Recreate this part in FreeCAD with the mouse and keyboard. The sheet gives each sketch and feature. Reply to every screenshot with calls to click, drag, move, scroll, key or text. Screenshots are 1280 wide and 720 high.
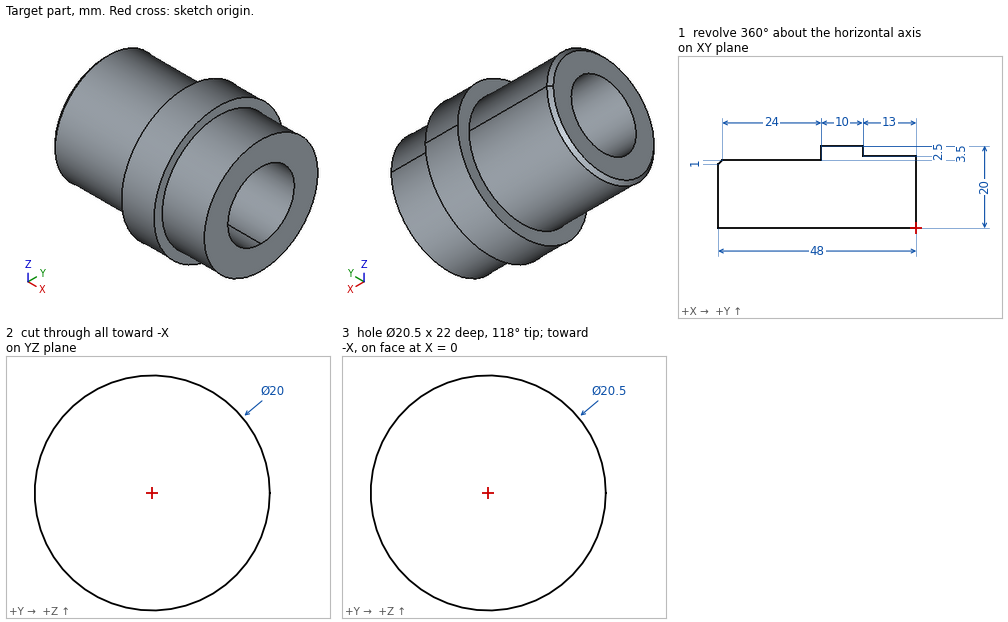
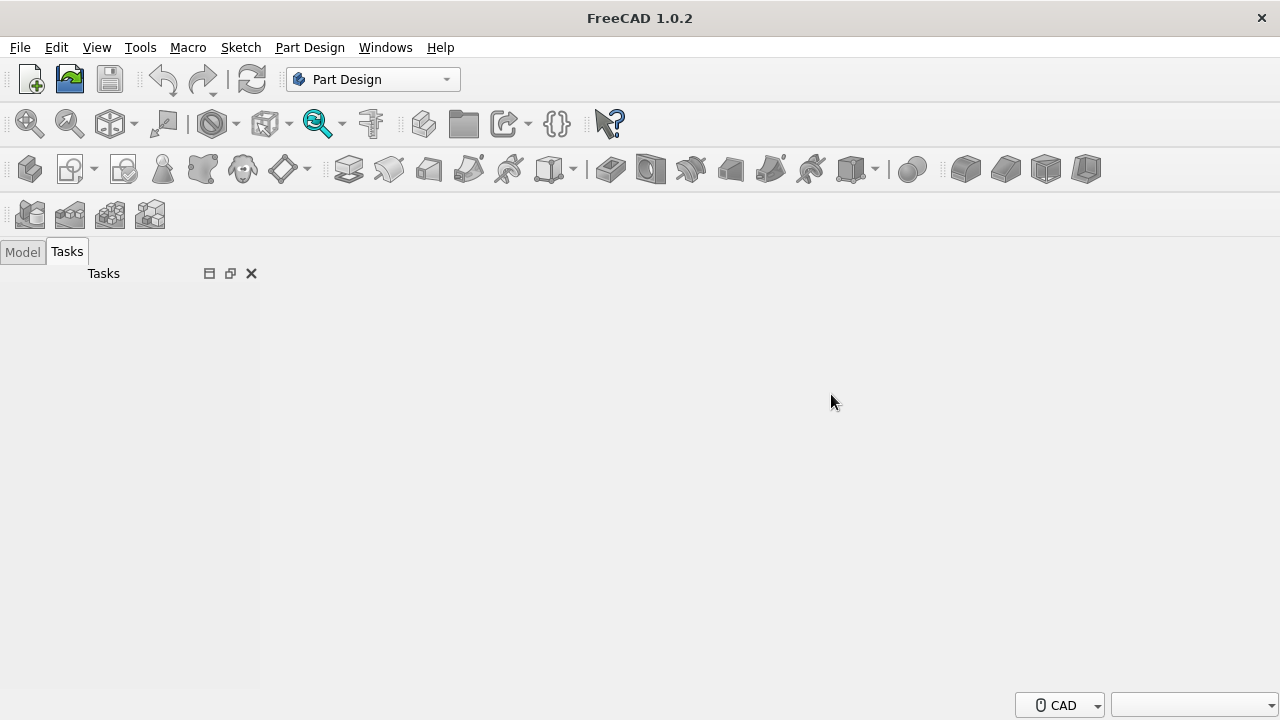
key(ctrl+n)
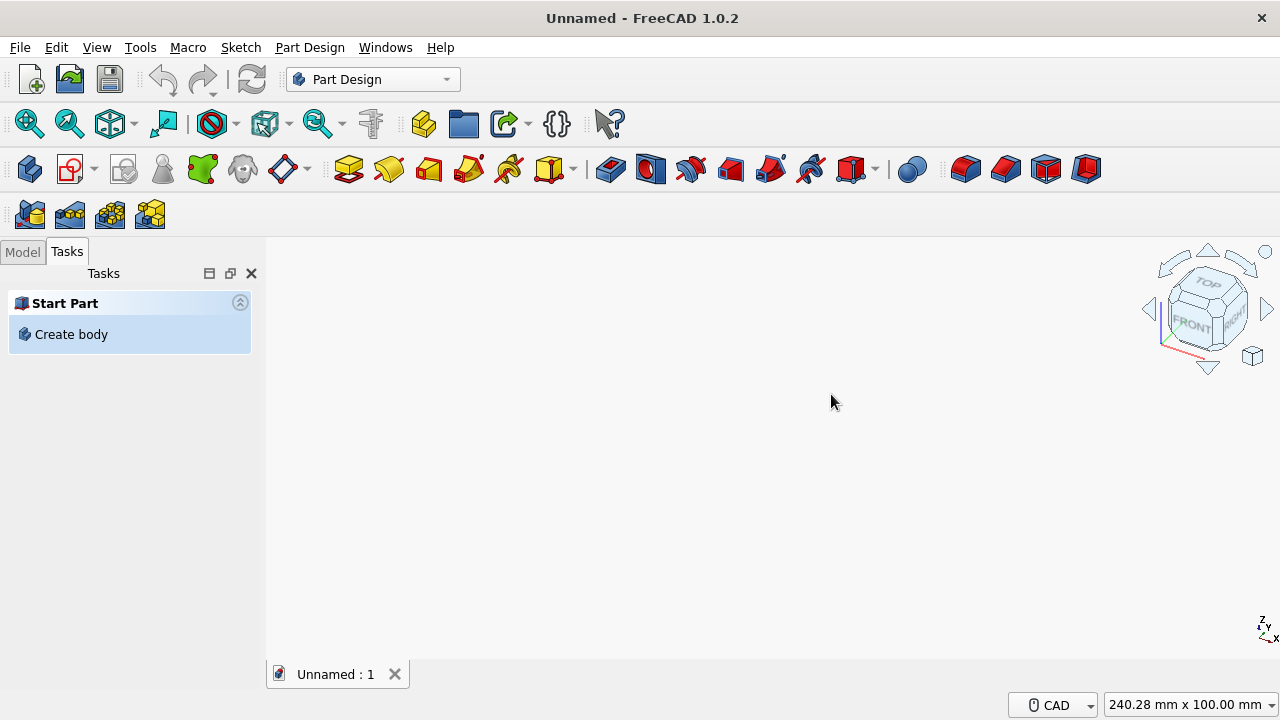
click(70, 170)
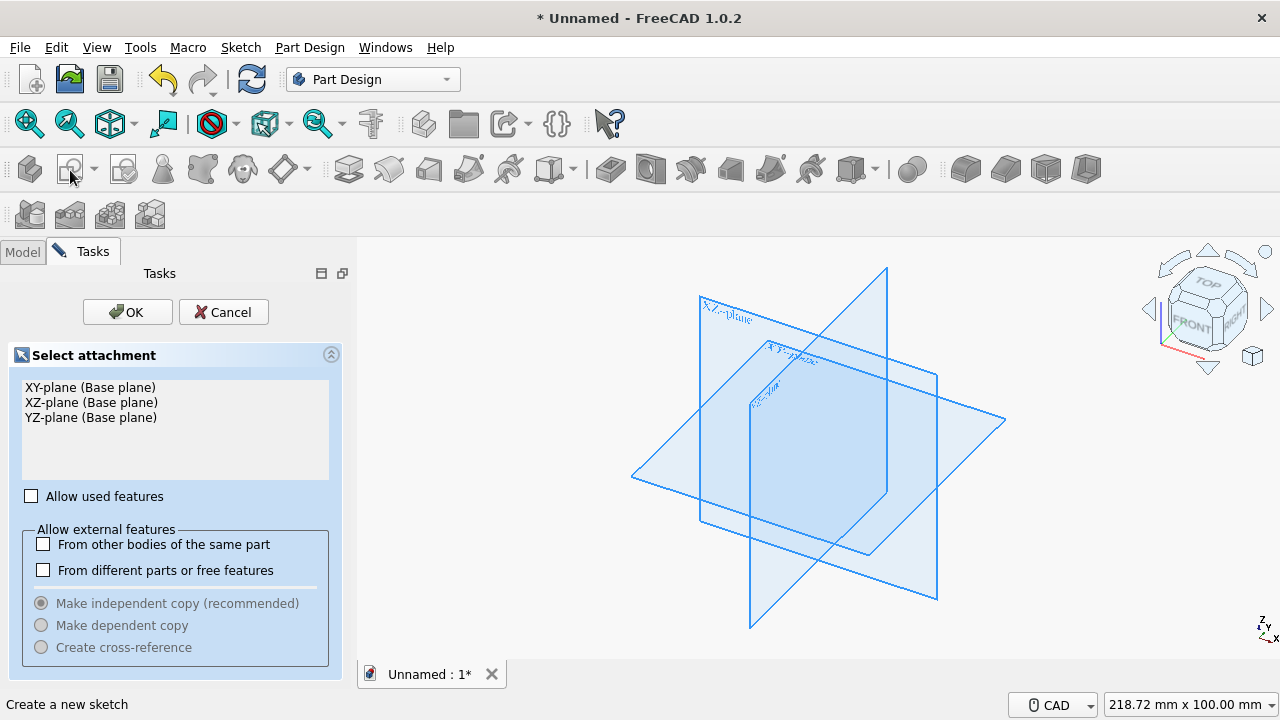
click(82, 388)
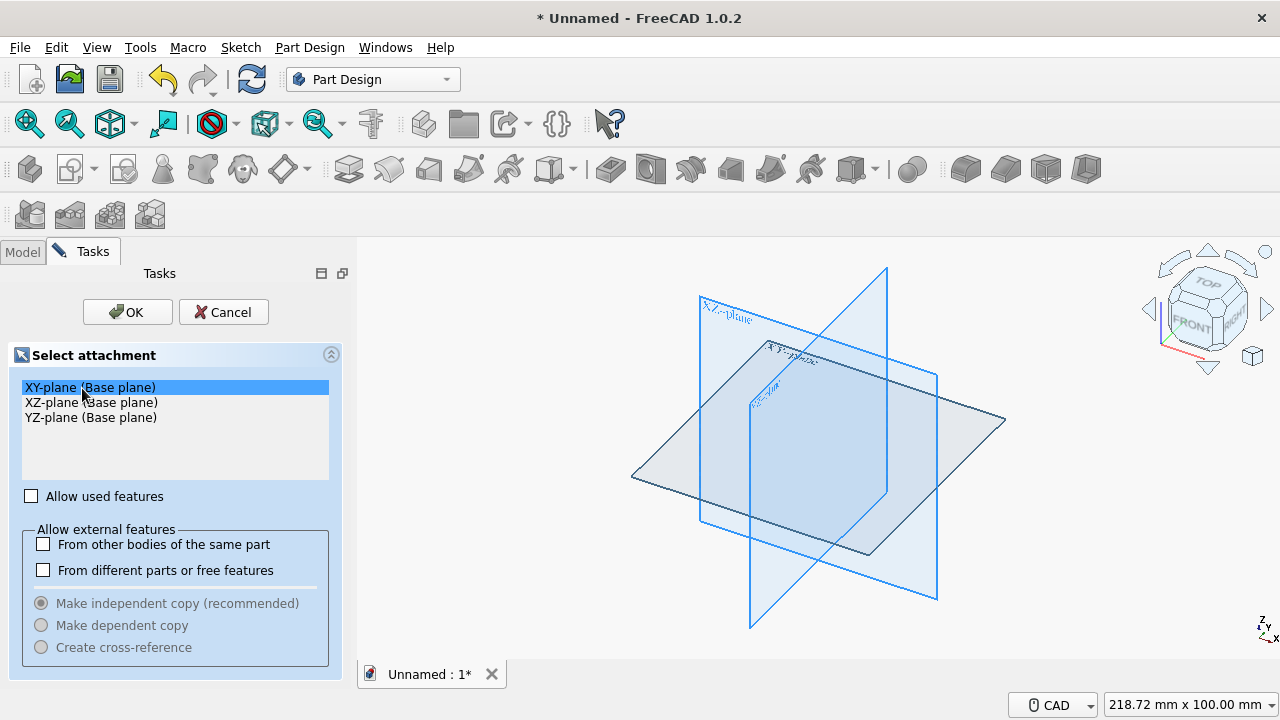
click(128, 312)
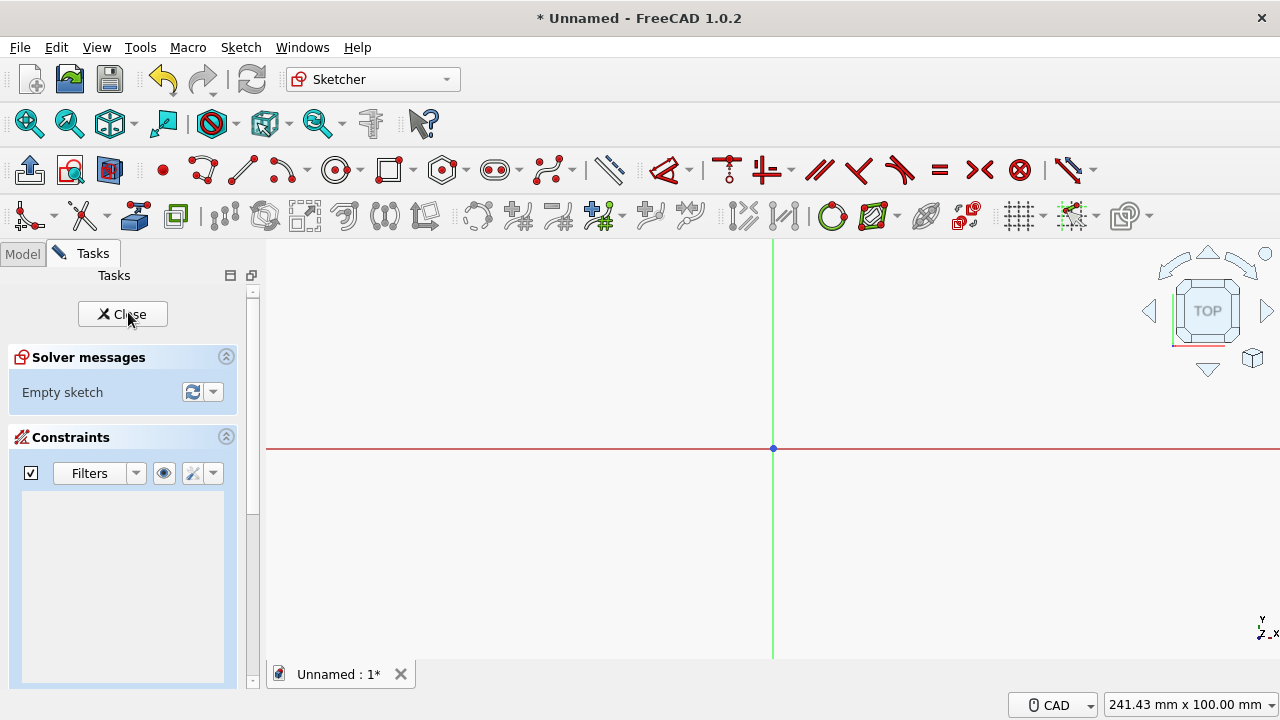
scroll(653, 383, up, 5)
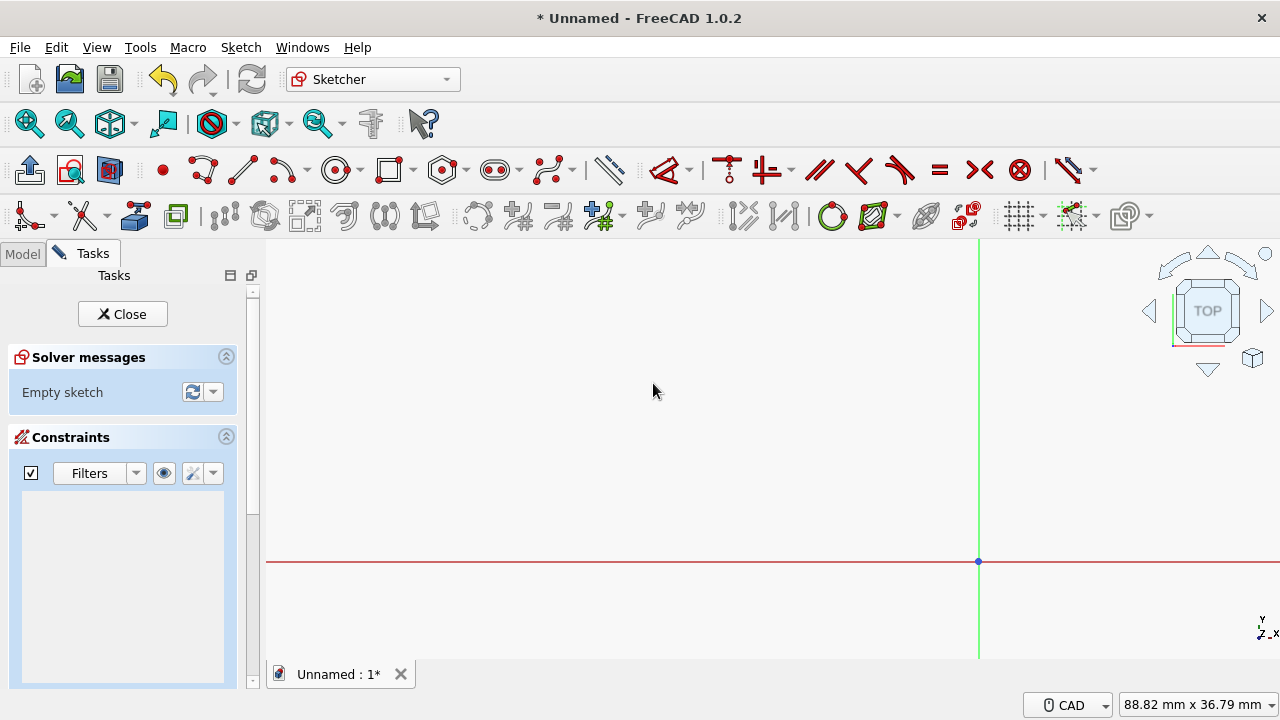
key(g)
key(m)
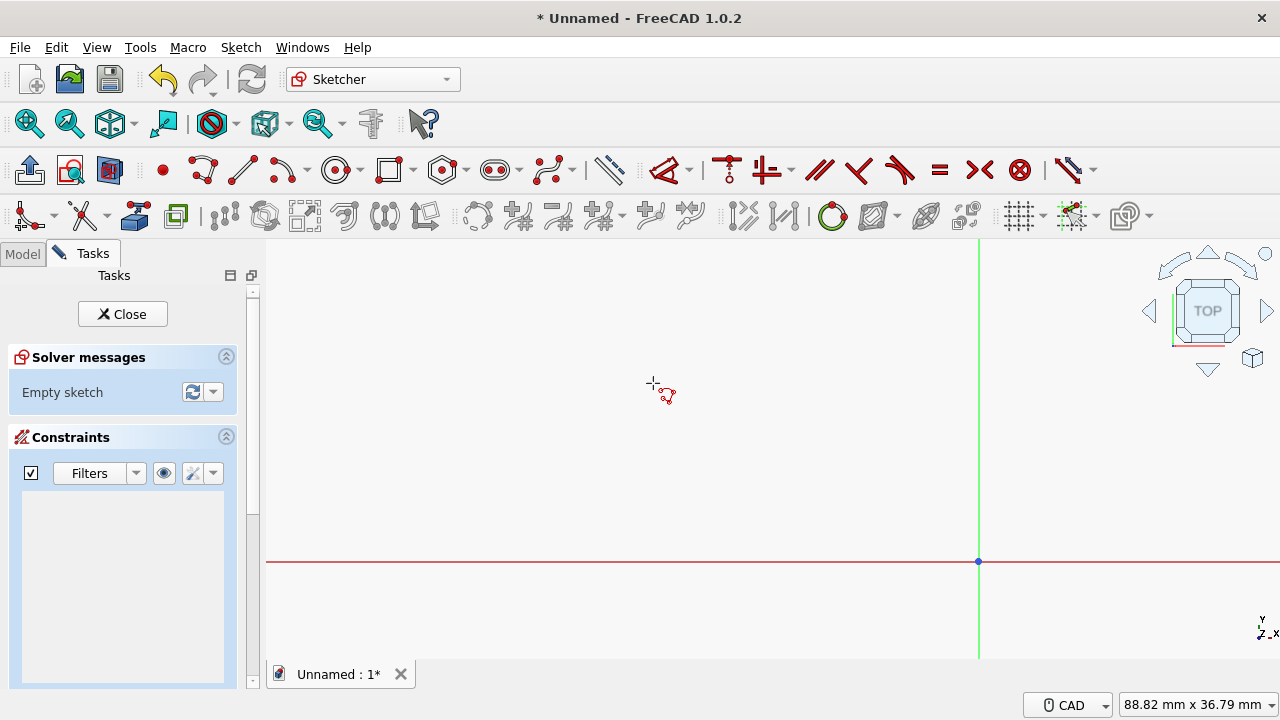
click(979, 562)
click(970, 362)
click(830, 362)
click(830, 333)
click(716, 333)
click(716, 373)
click(442, 373)
click(431, 385)
click(431, 553)
click(979, 562)
key(Escape)
key(Escape)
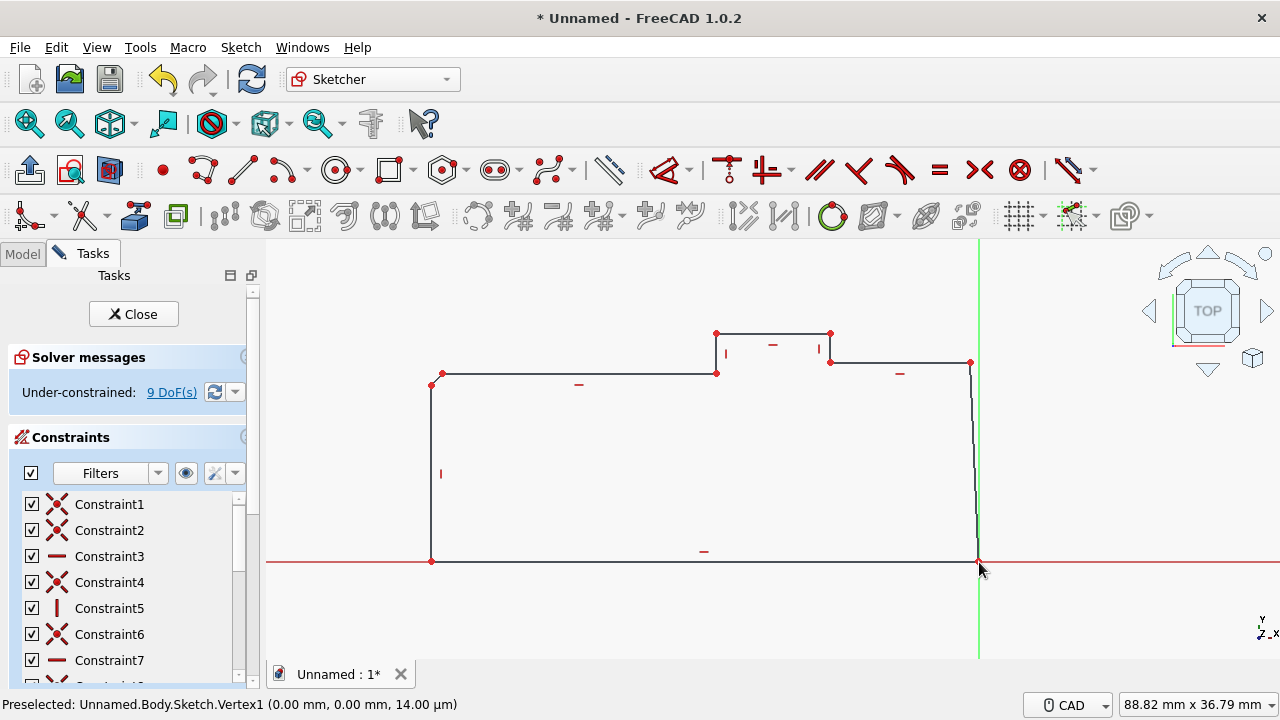
click(976, 502)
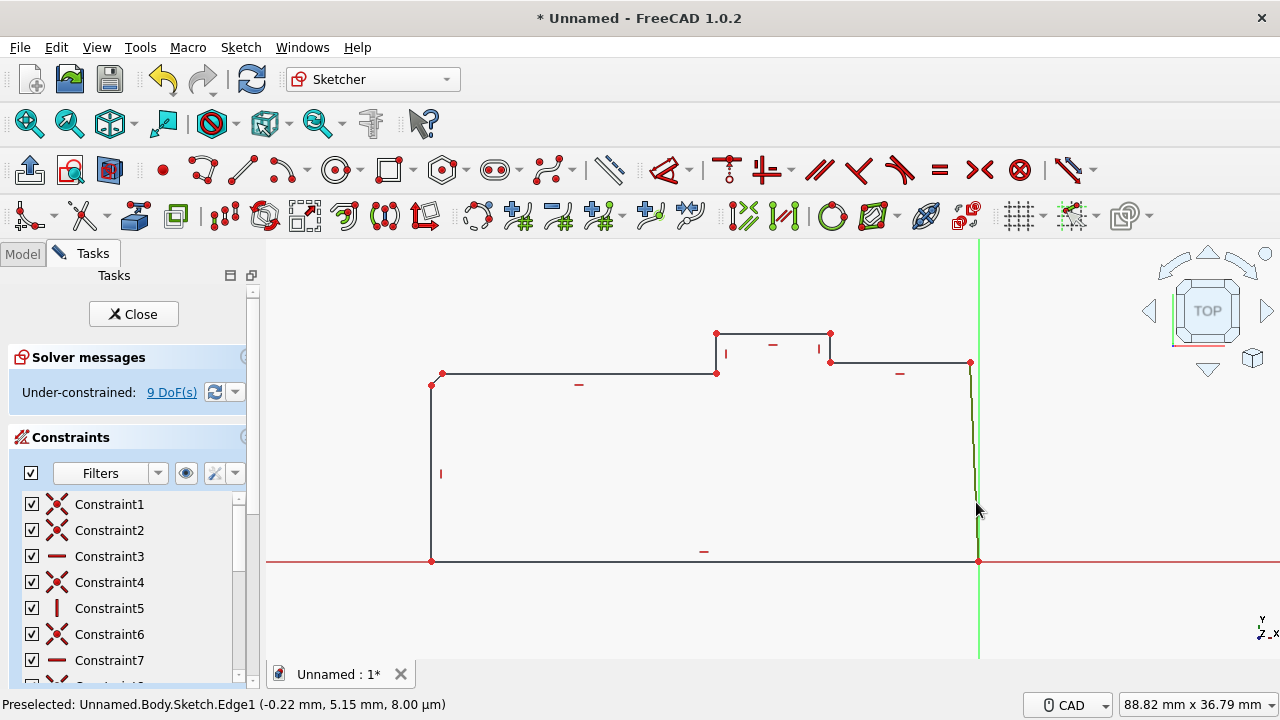
key(v)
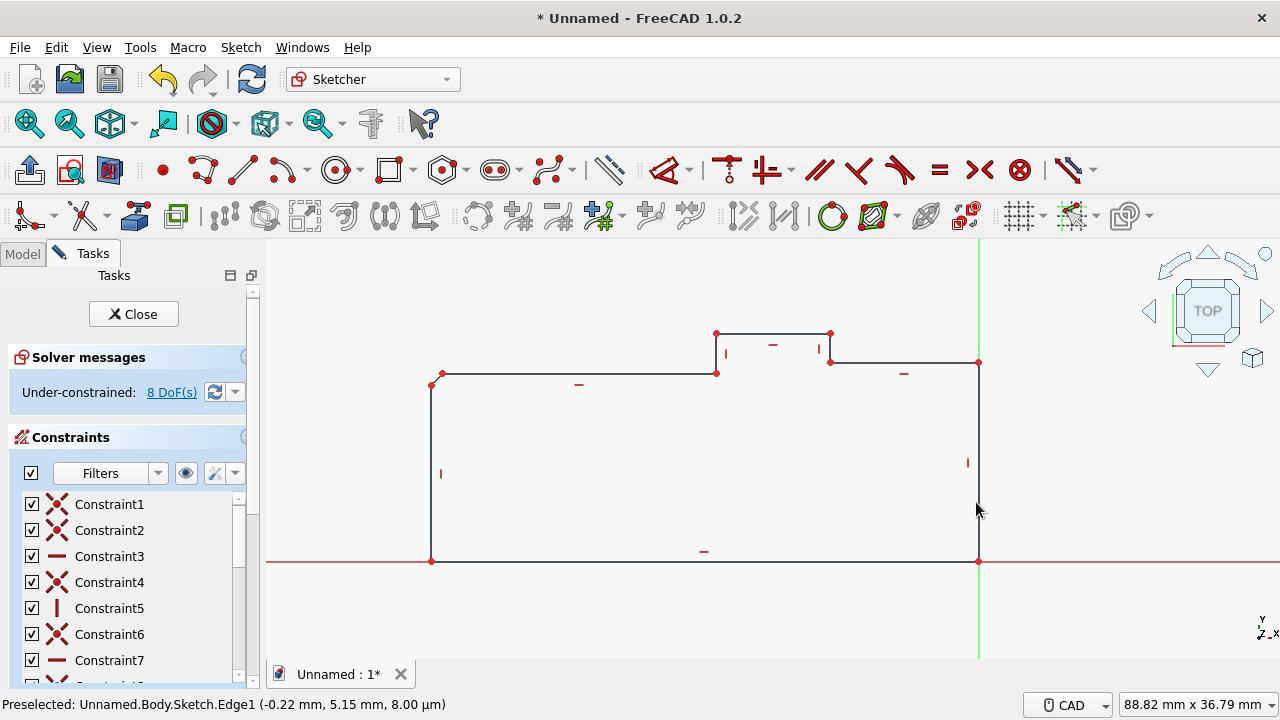
key(d)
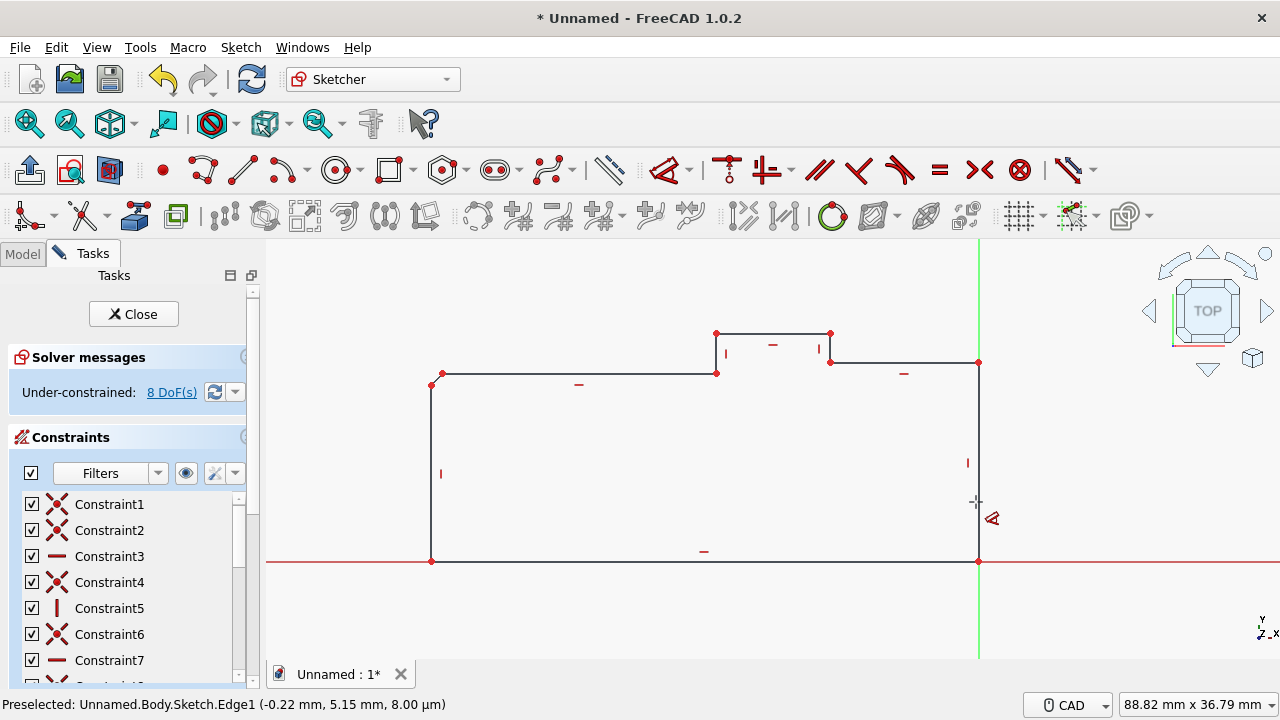
click(934, 363)
click(904, 329)